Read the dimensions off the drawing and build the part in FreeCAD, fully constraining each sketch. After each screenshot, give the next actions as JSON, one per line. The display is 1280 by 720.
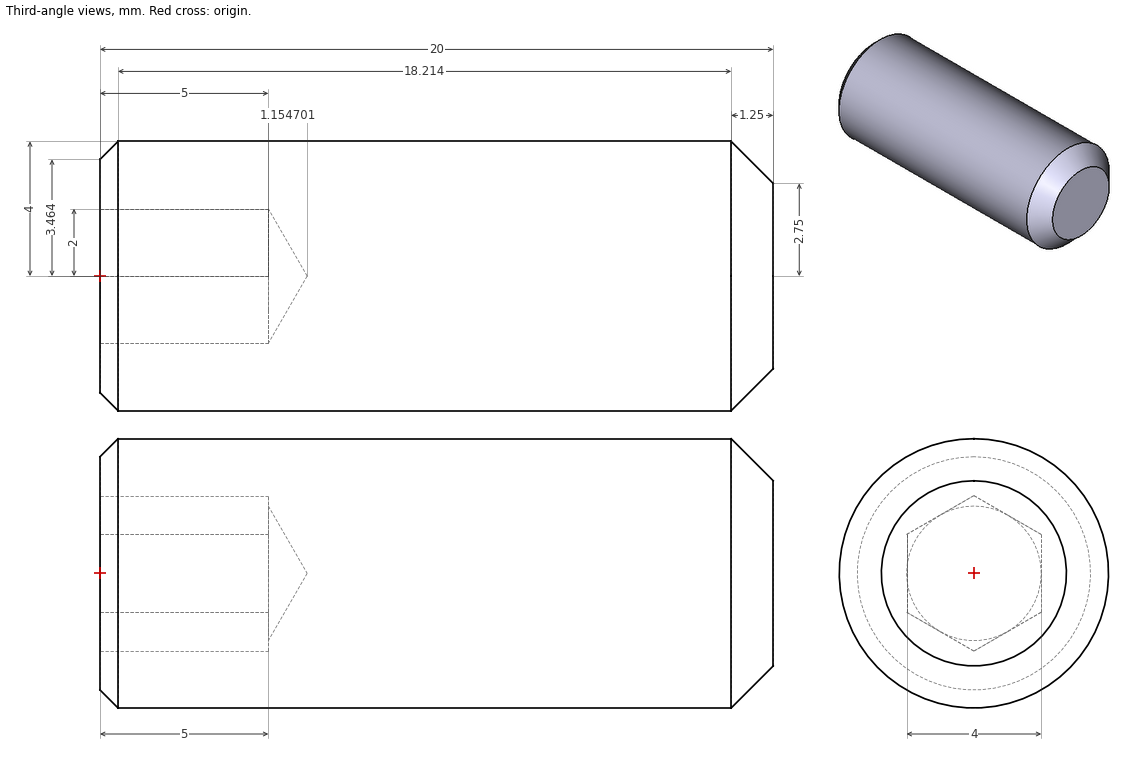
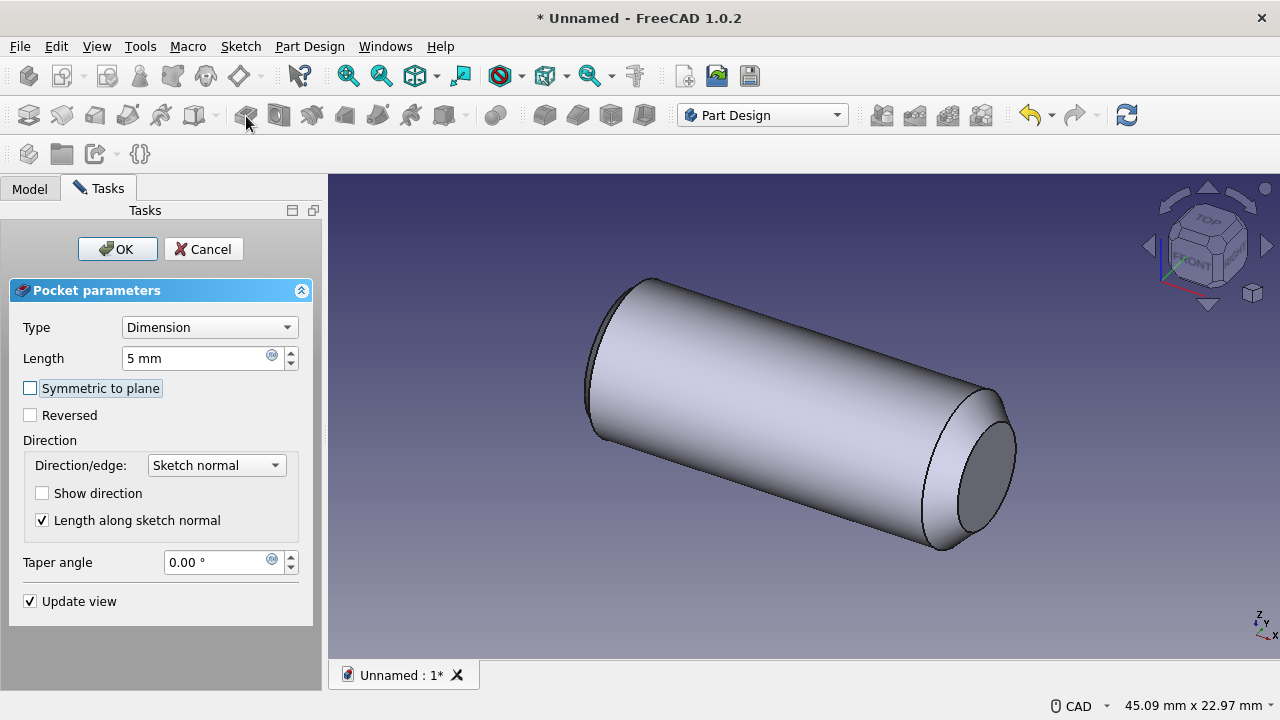
{"action": "left_click", "coordinate": [31, 415]}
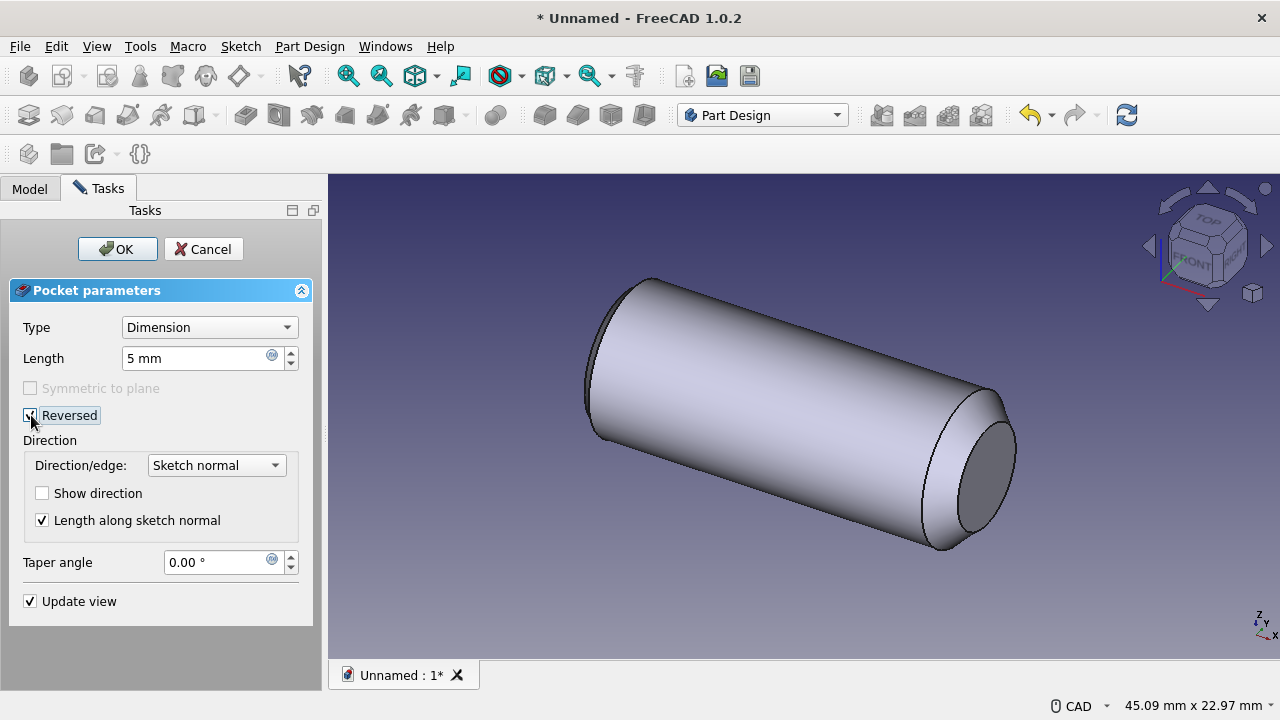
{"action": "left_click", "coordinate": [118, 249]}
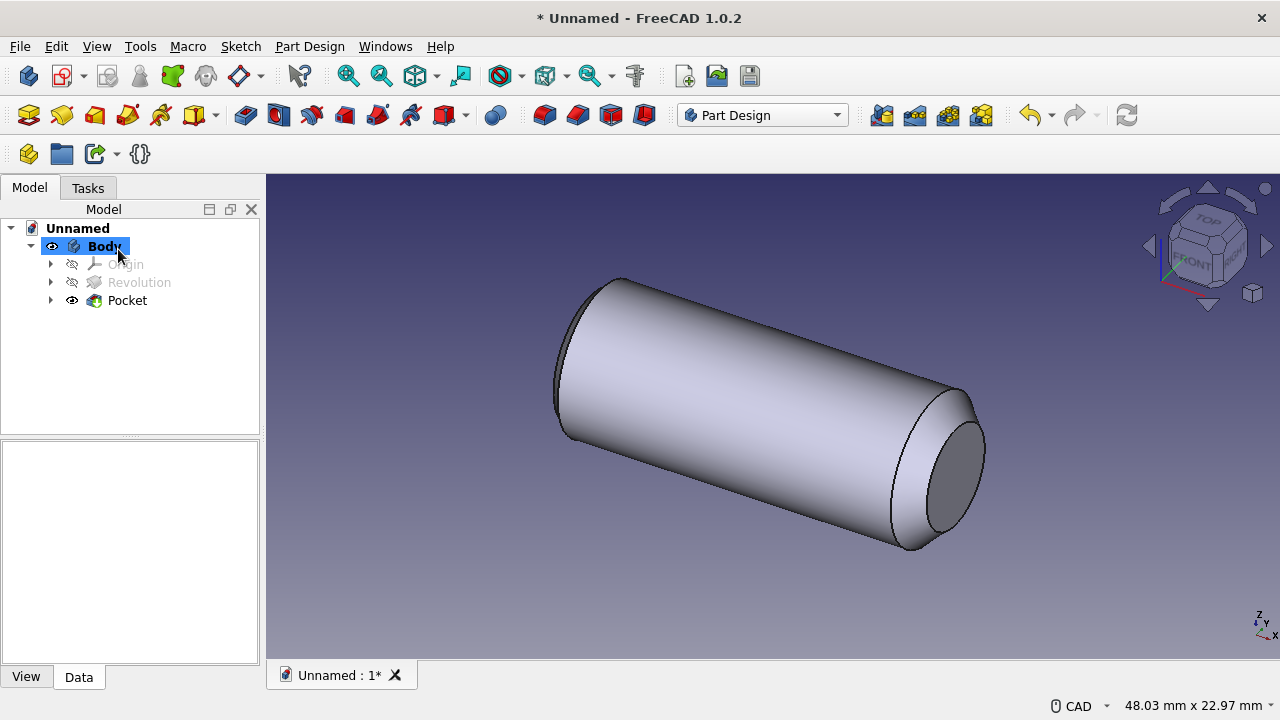
{"action": "left_click", "coordinate": [62, 76]}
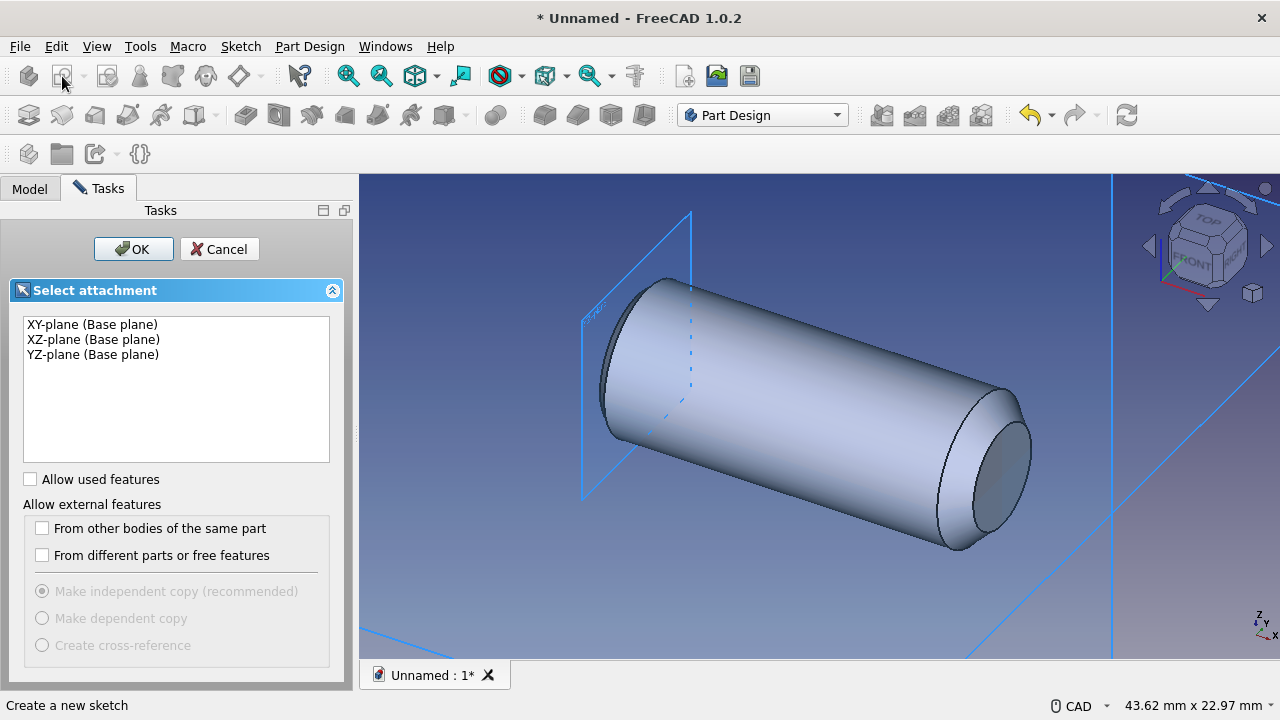
{"action": "left_click", "coordinate": [84, 324]}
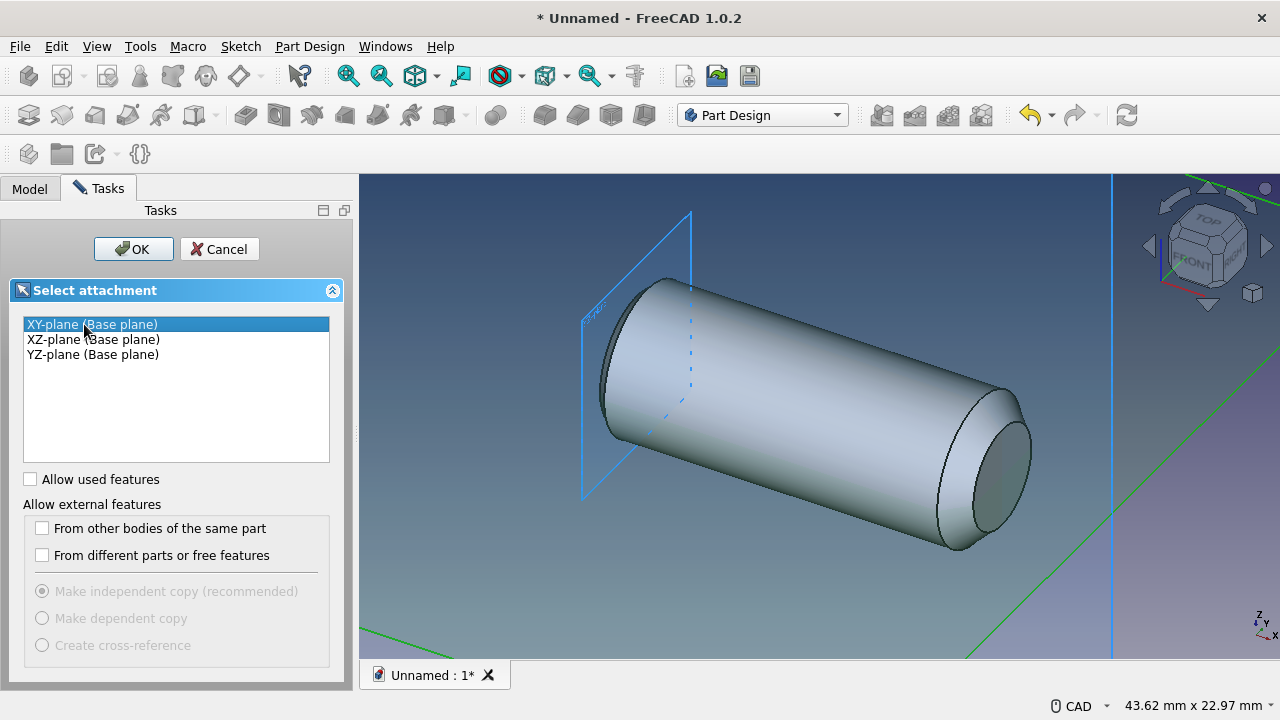
{"action": "left_click", "coordinate": [134, 249]}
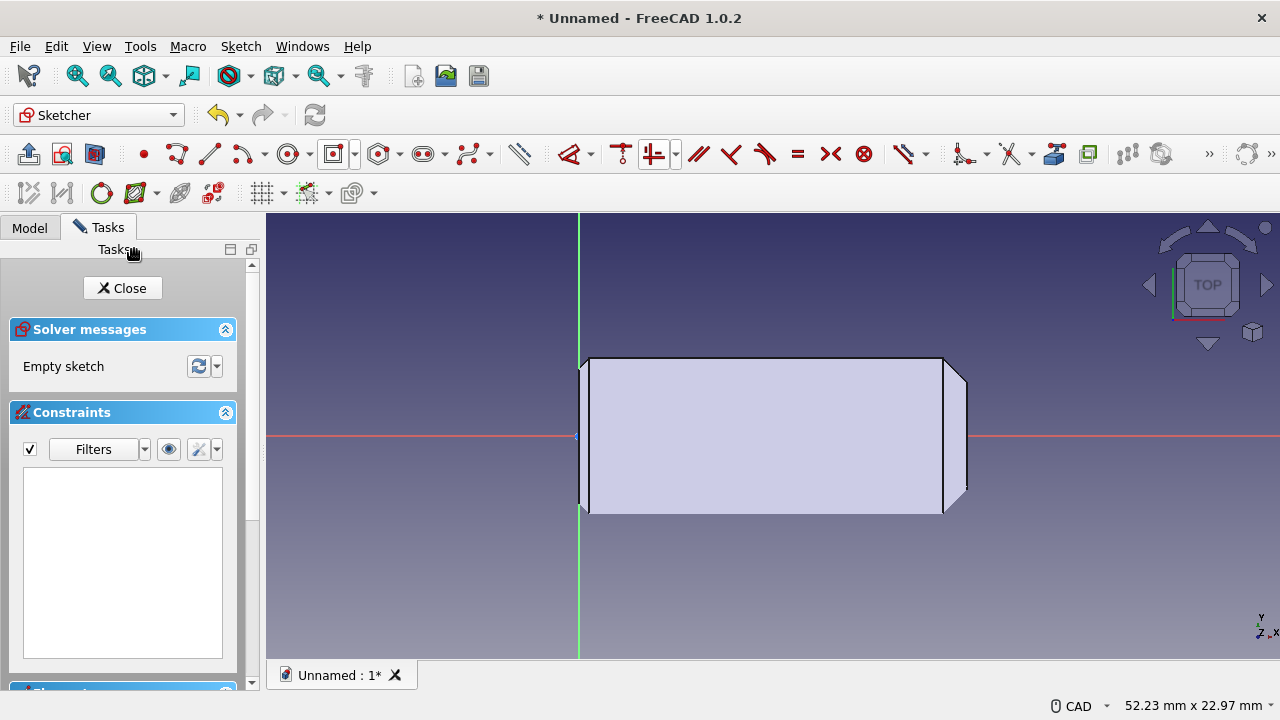
{"action": "key", "text": "q s"}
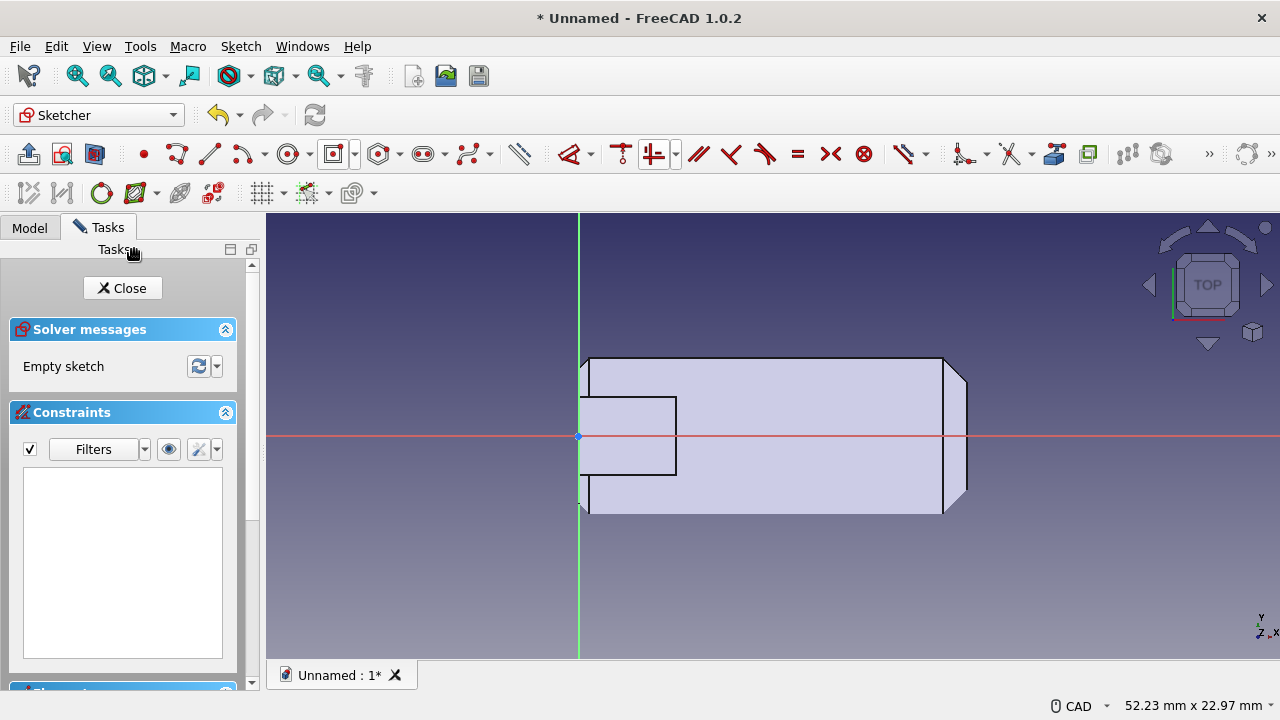
{"action": "scroll", "coordinate": [684, 414], "scroll_direction": "up", "scroll_amount": 10}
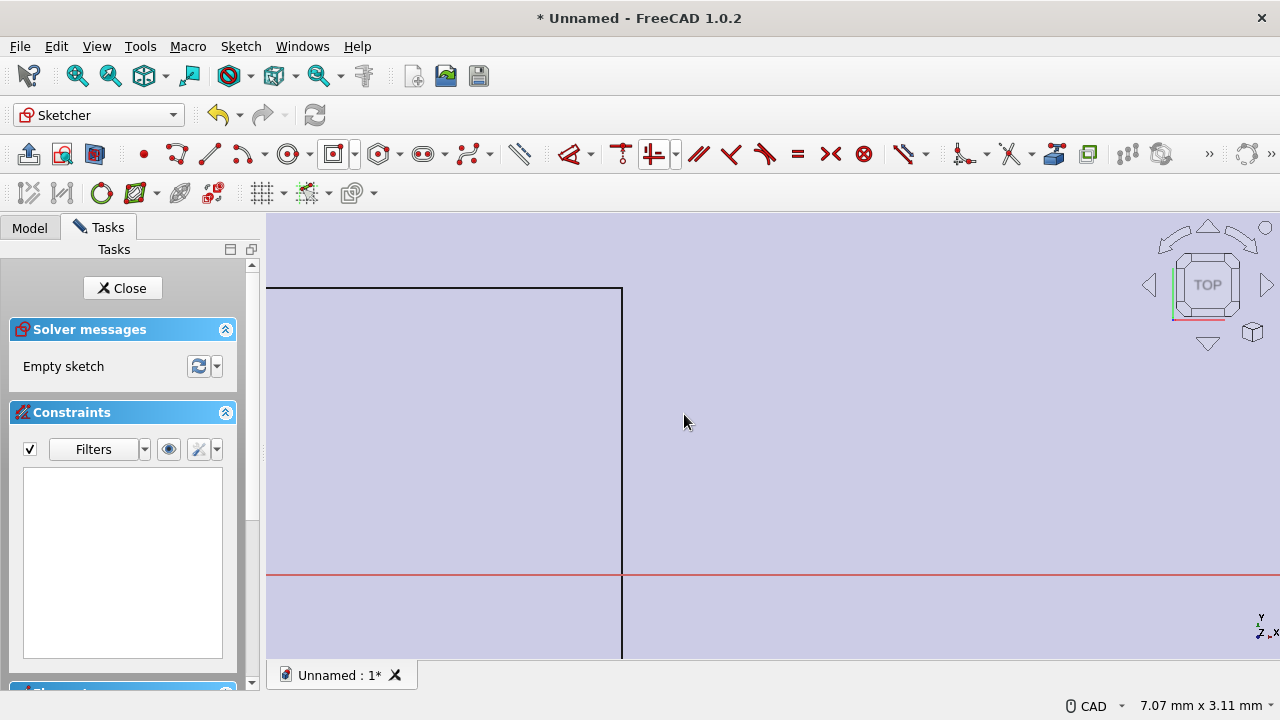
{"action": "left_click", "coordinate": [177, 154]}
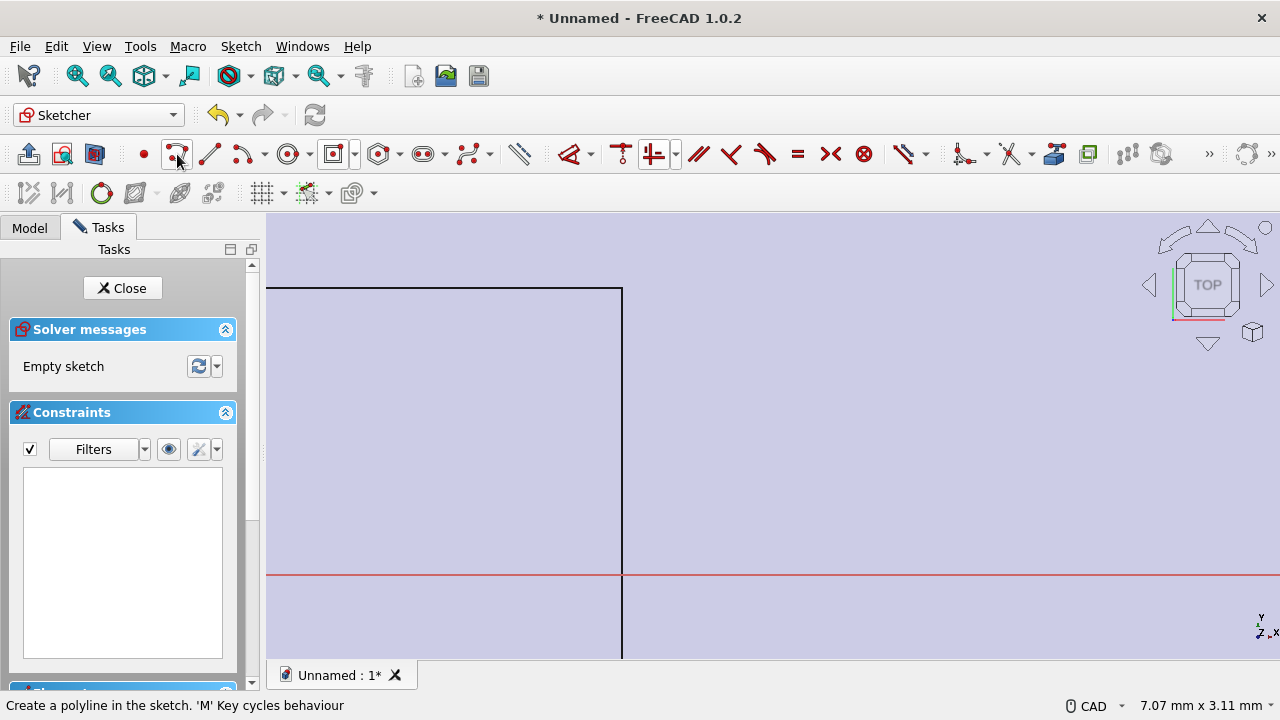
{"action": "left_click", "coordinate": [622, 575]}
{"action": "left_click", "coordinate": [787, 566]}
{"action": "left_click", "coordinate": [622, 288]}
{"action": "left_click", "coordinate": [622, 575]}
{"action": "key", "text": "Escape"}
{"action": "key", "text": "Escape"}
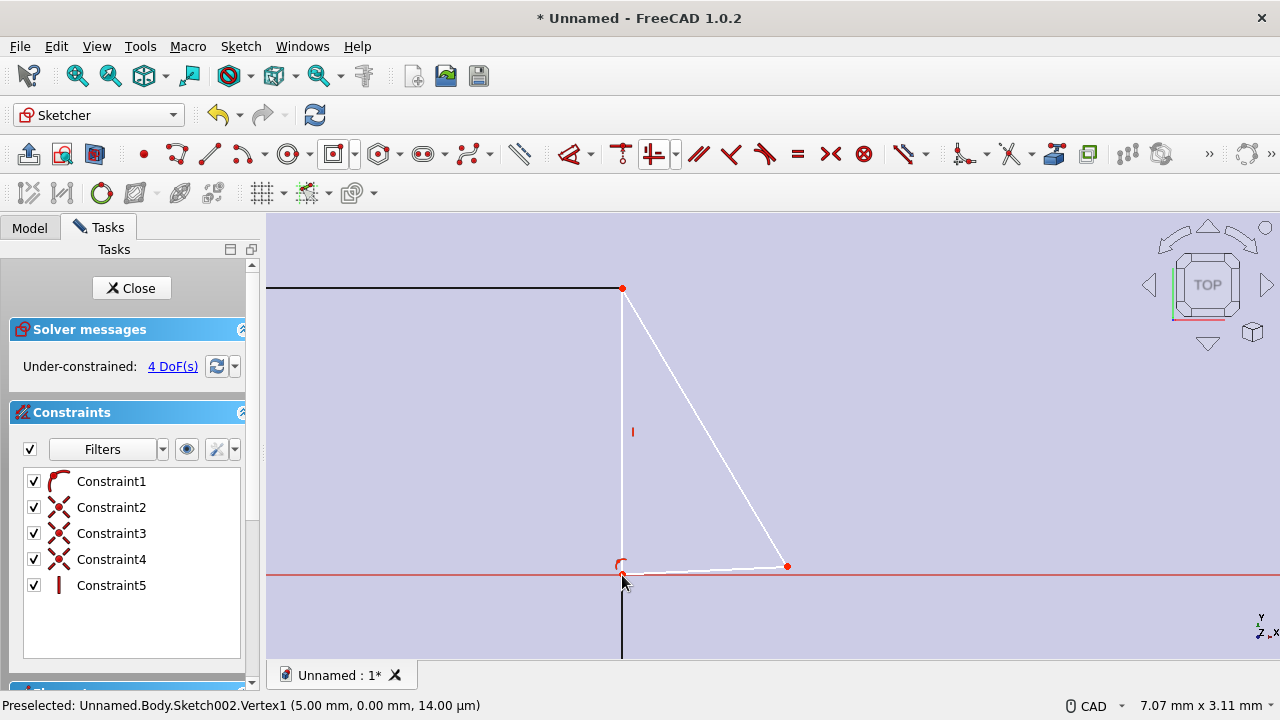
{"action": "left_click", "coordinate": [671, 572]}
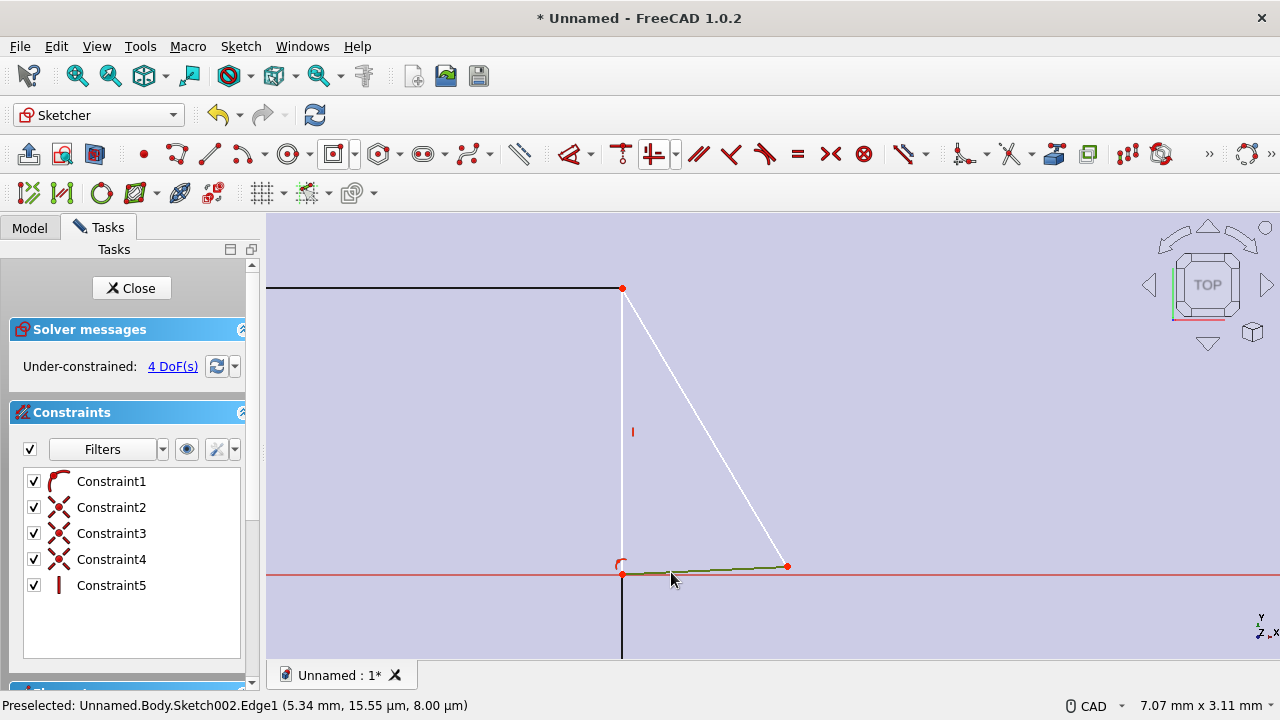
{"action": "key", "text": "h"}